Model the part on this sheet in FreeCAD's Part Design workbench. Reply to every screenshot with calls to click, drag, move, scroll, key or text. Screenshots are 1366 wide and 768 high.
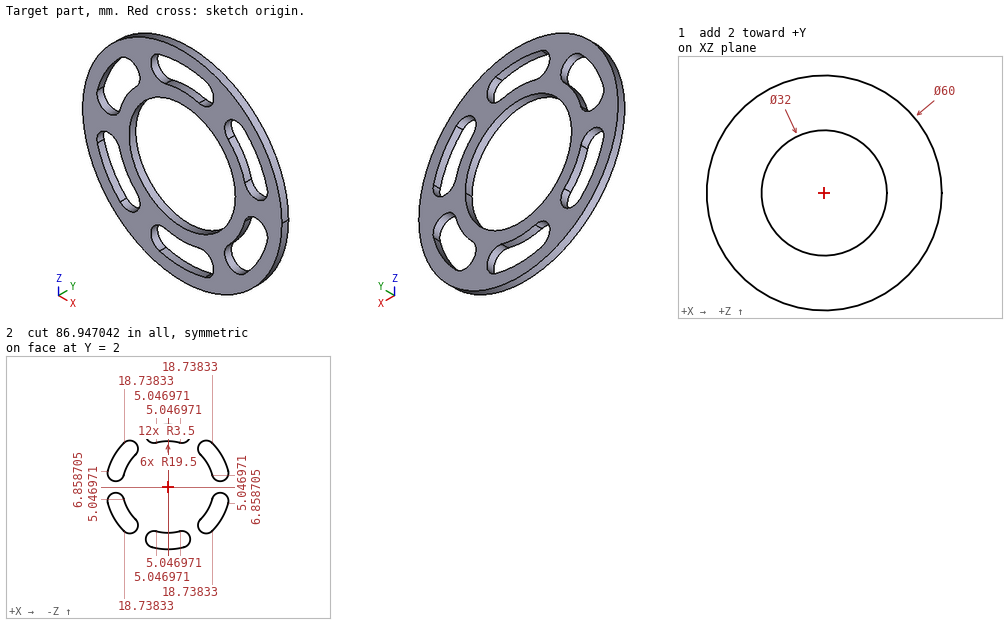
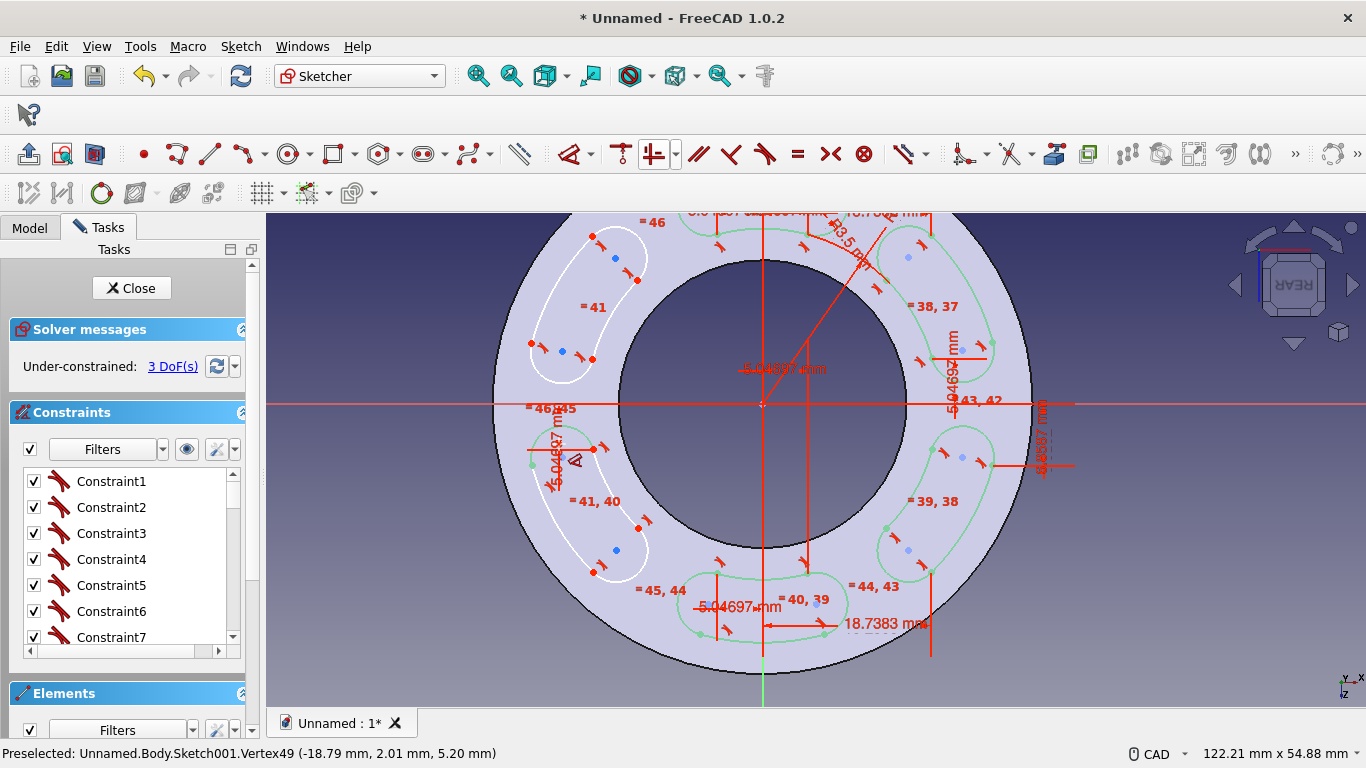
click(594, 573)
click(639, 607)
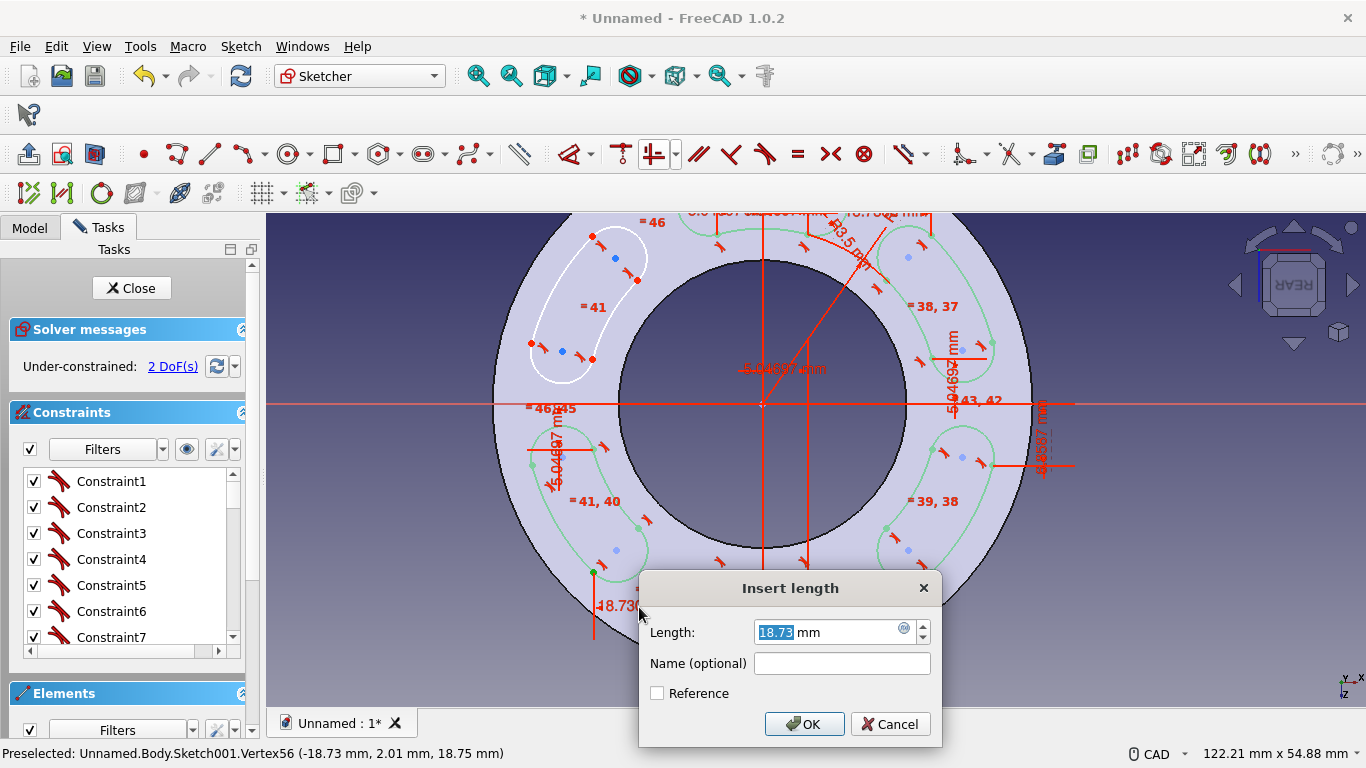
text(18.73833)
key(Return)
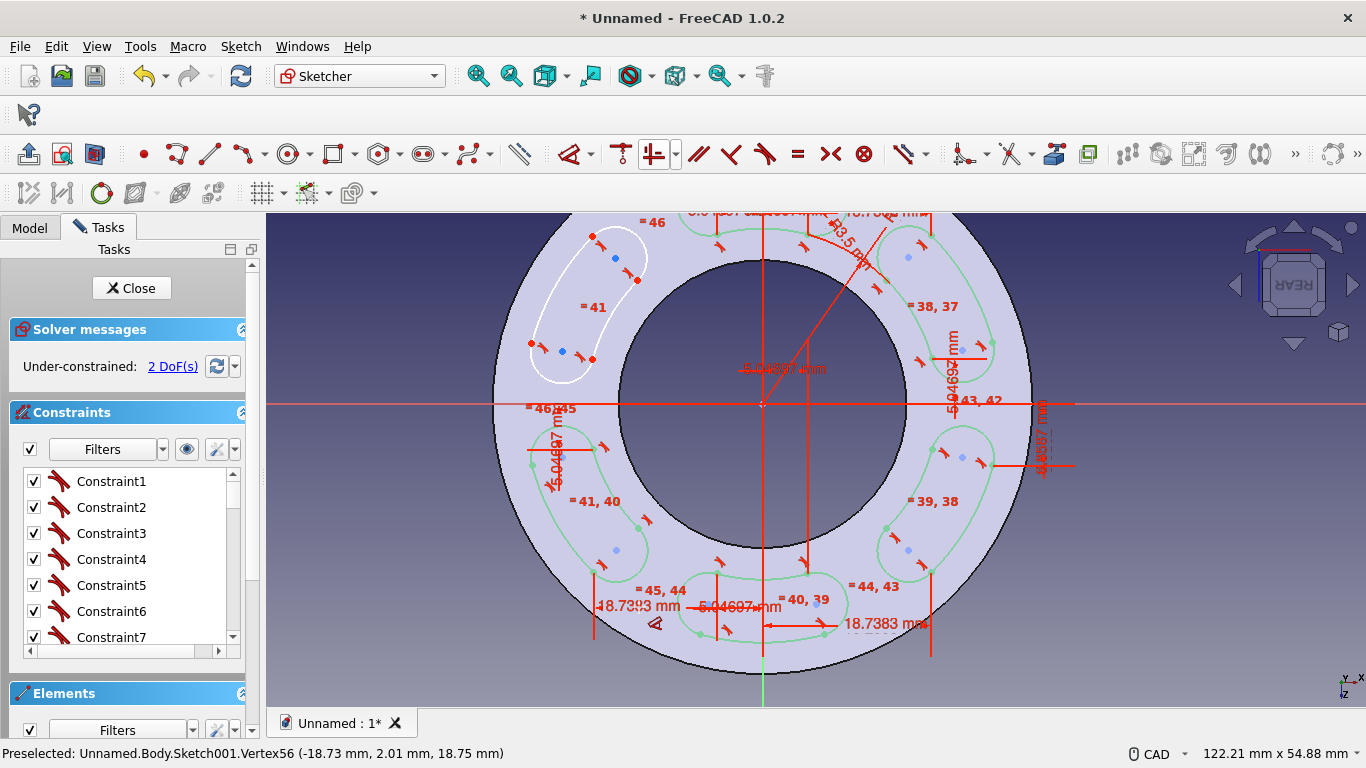
scroll(717, 574, down, 2)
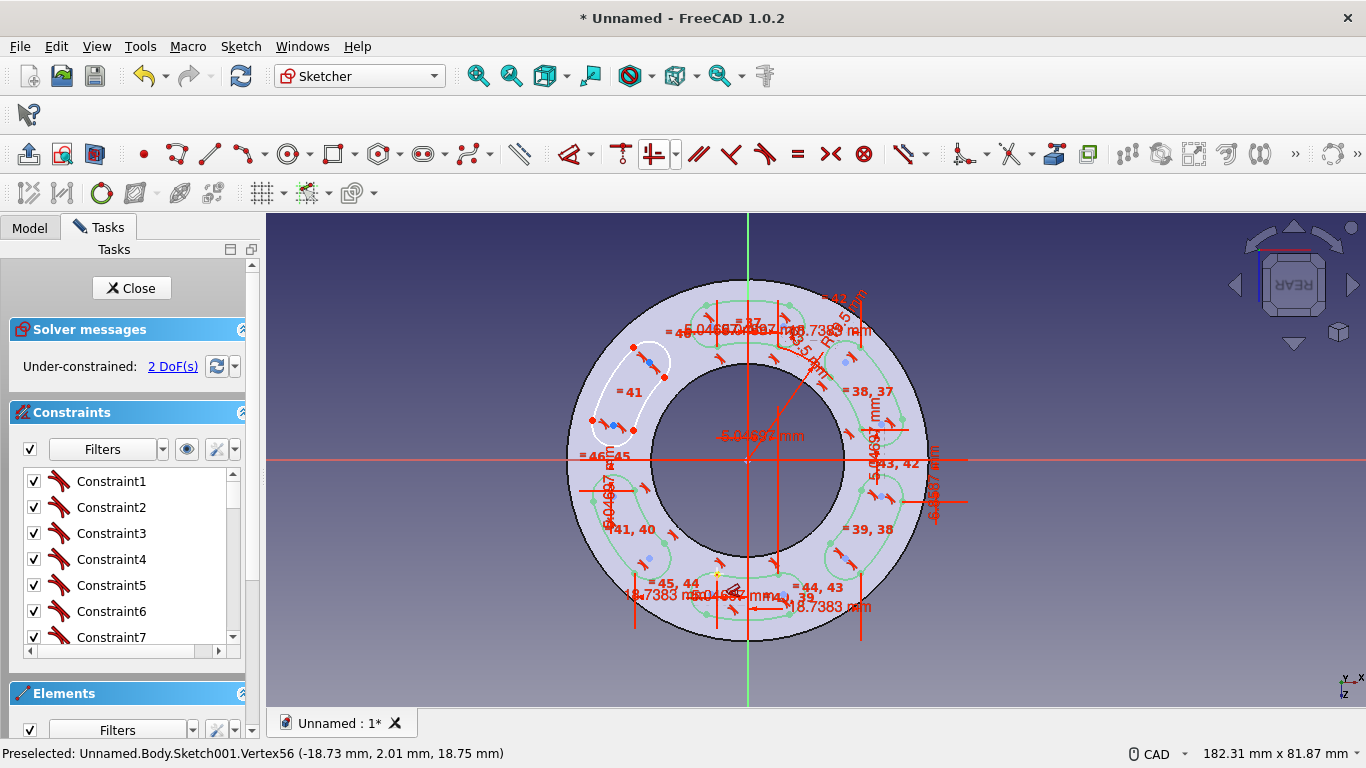
click(634, 348)
click(651, 314)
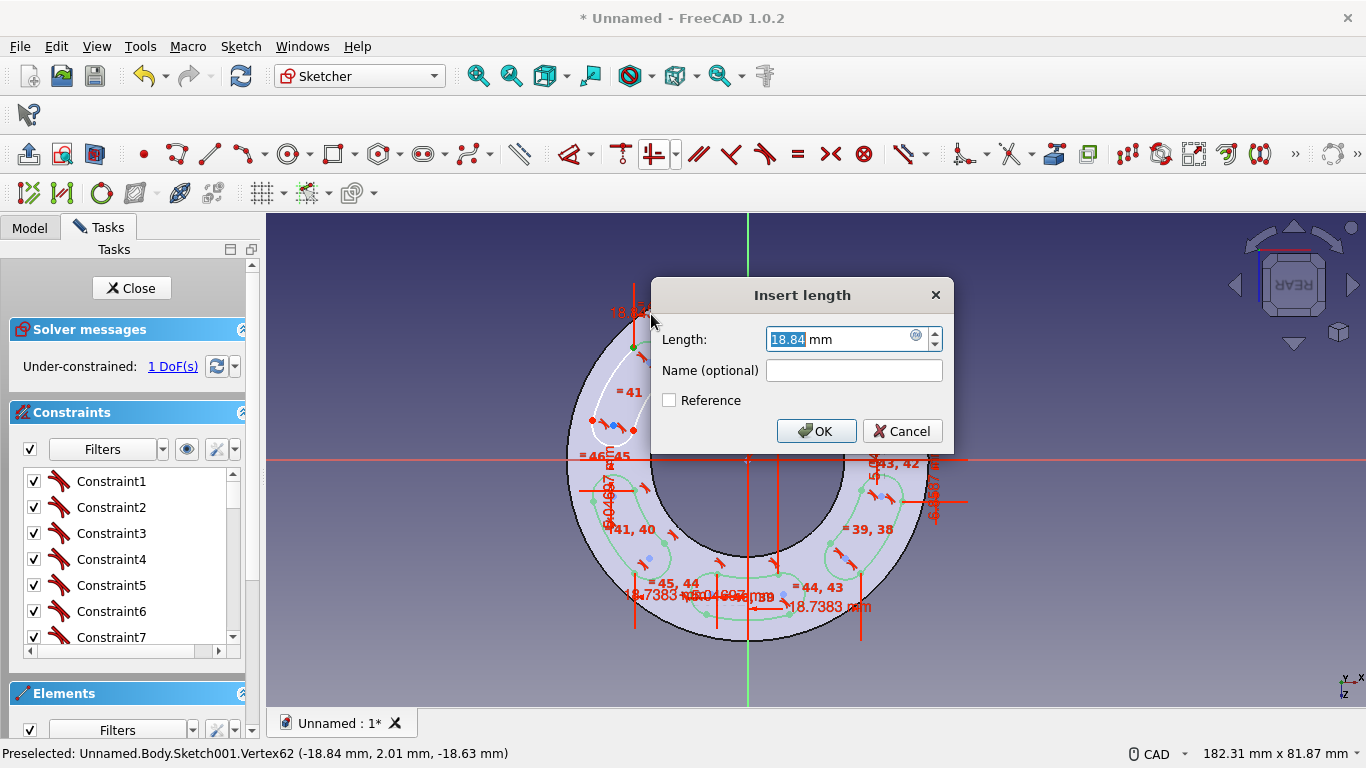
text(18.73833)
key(Return)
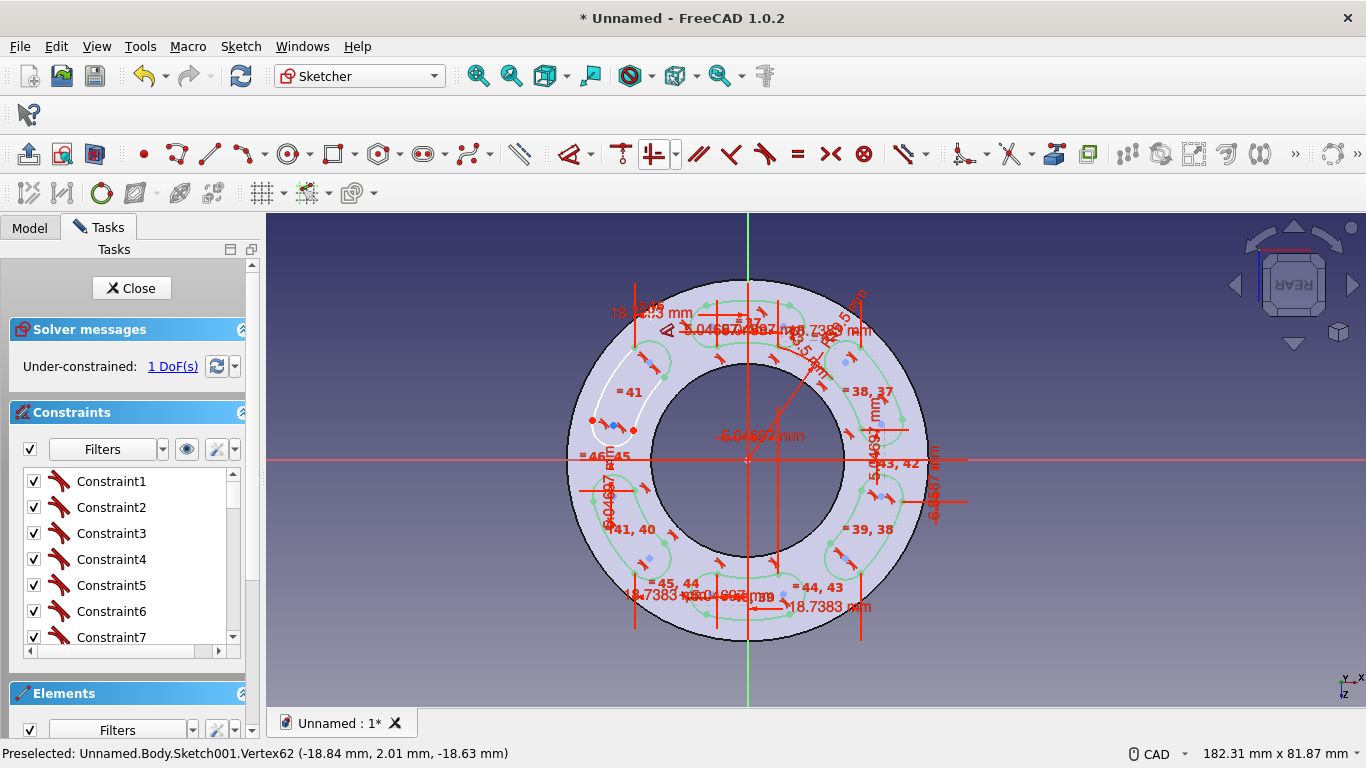
click(593, 420)
click(559, 440)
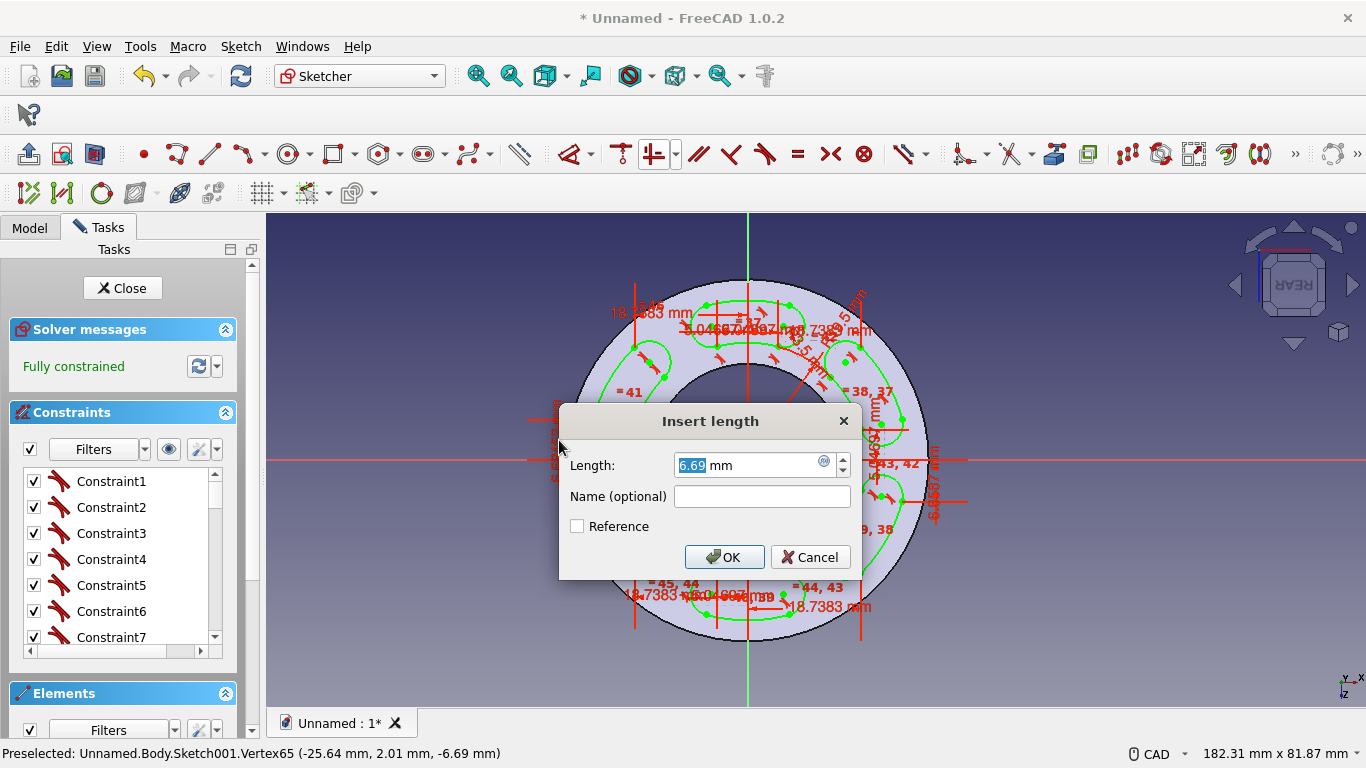
text(6.858705)
key(Return)
key(Escape)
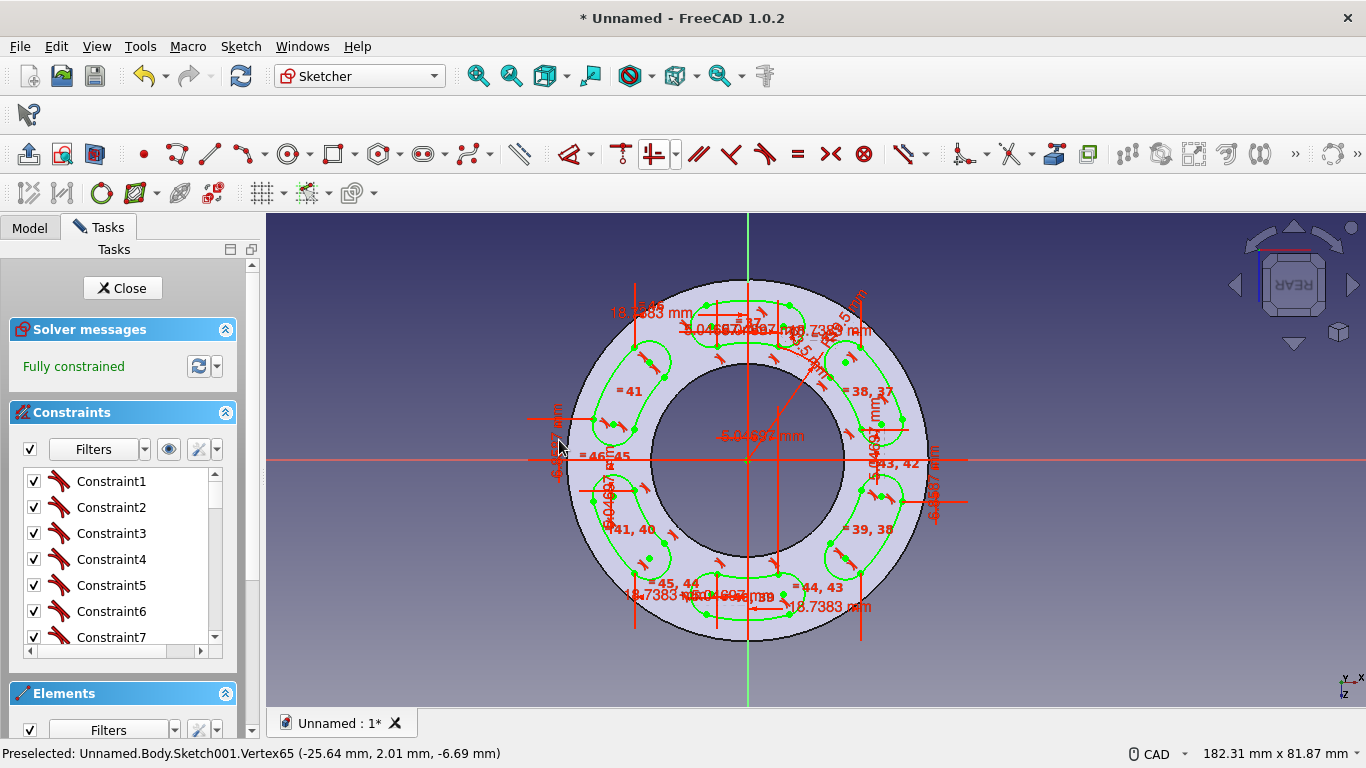
click(123, 288)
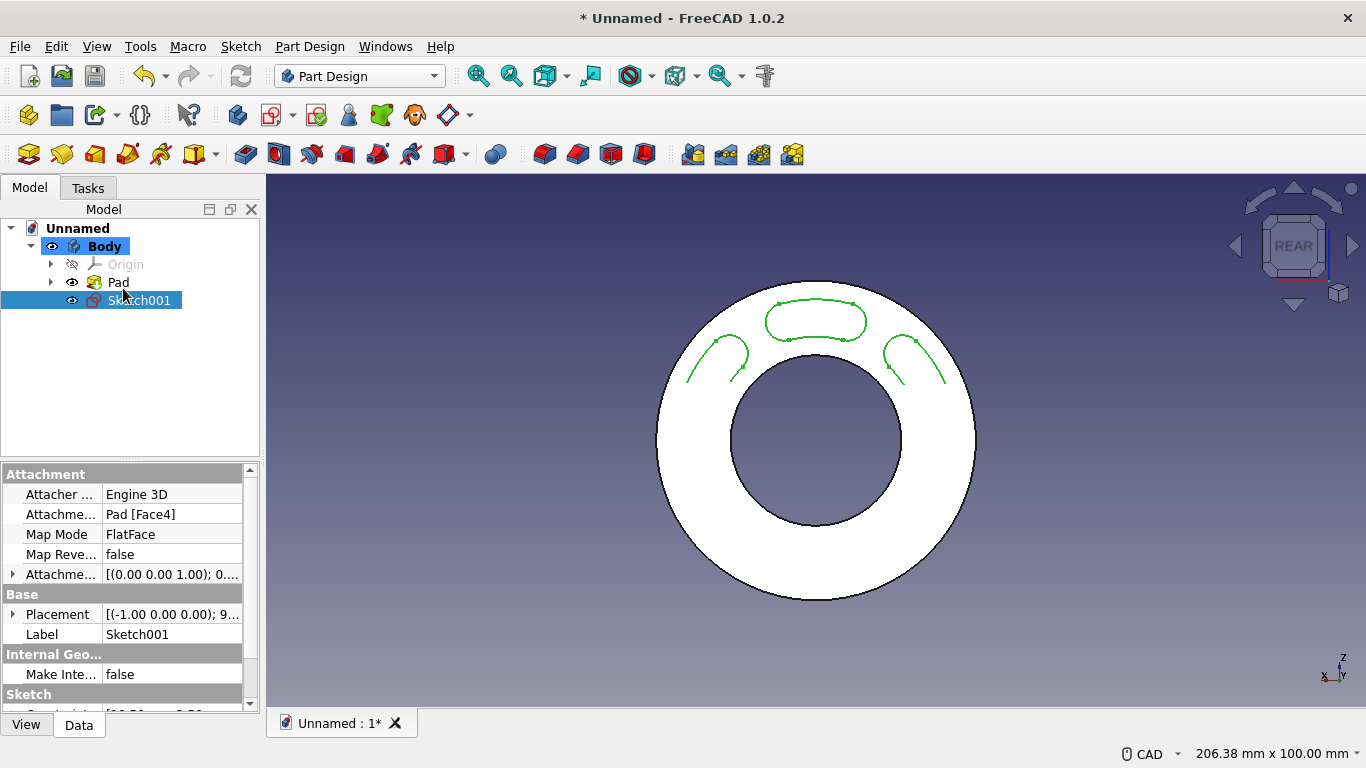
click(246, 154)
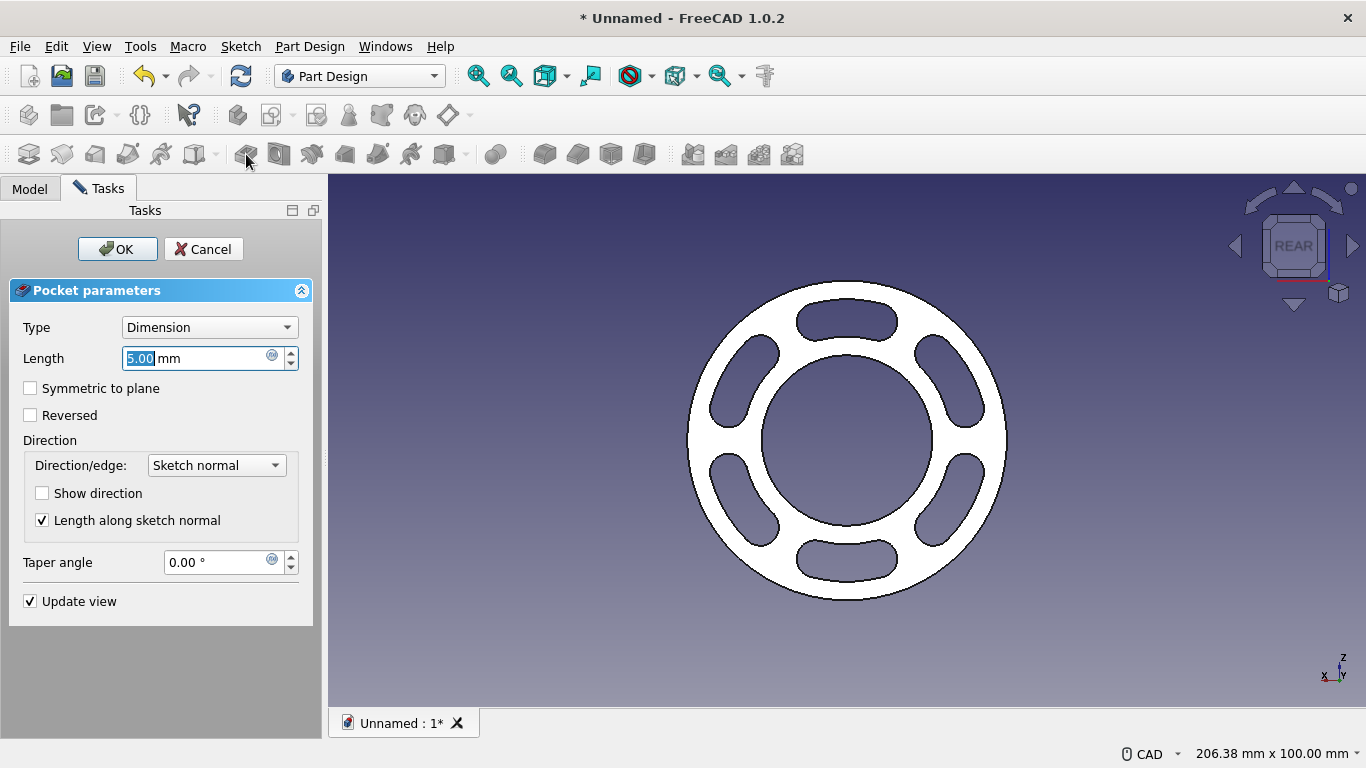
text(86.947042)
key(Tab)